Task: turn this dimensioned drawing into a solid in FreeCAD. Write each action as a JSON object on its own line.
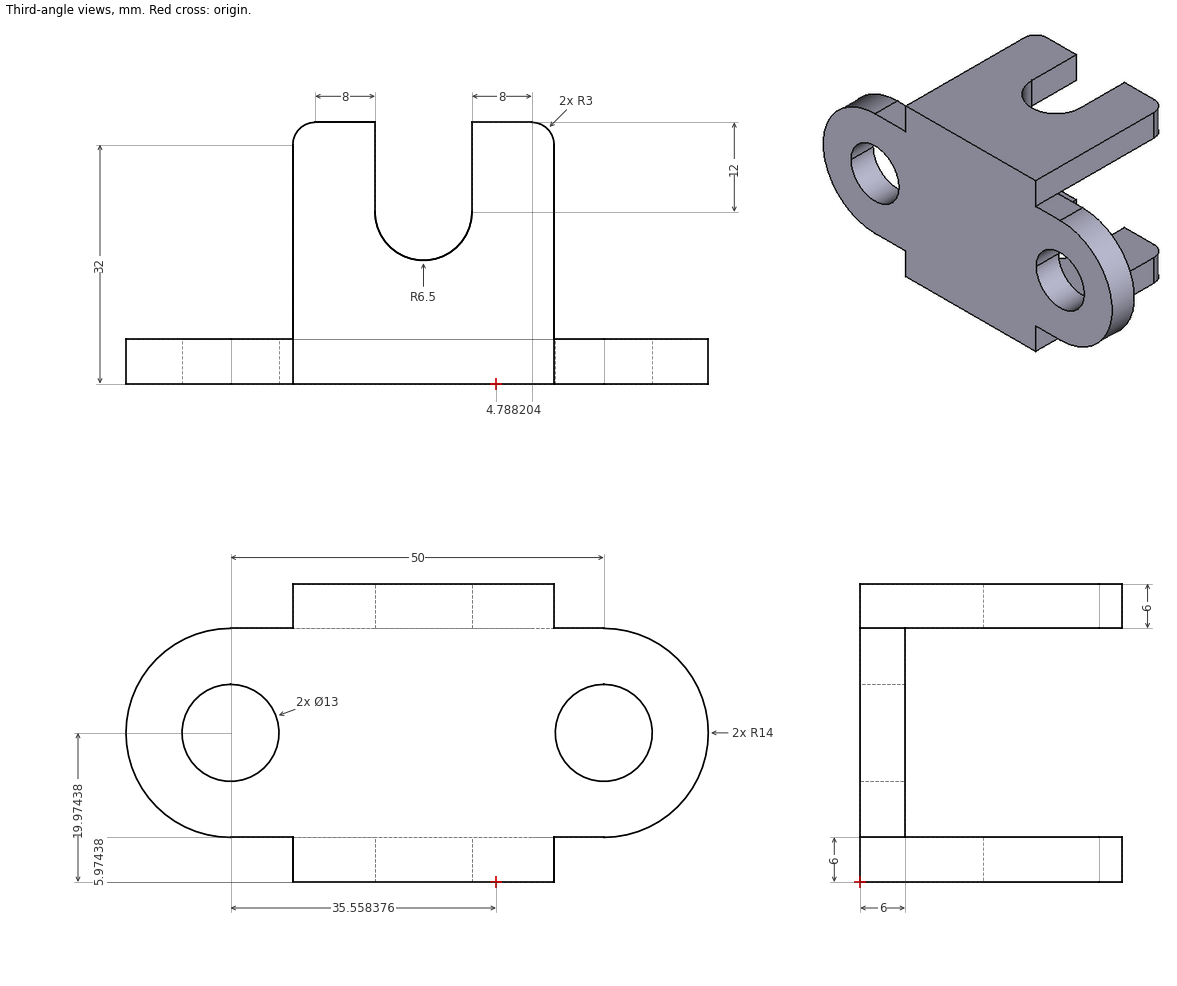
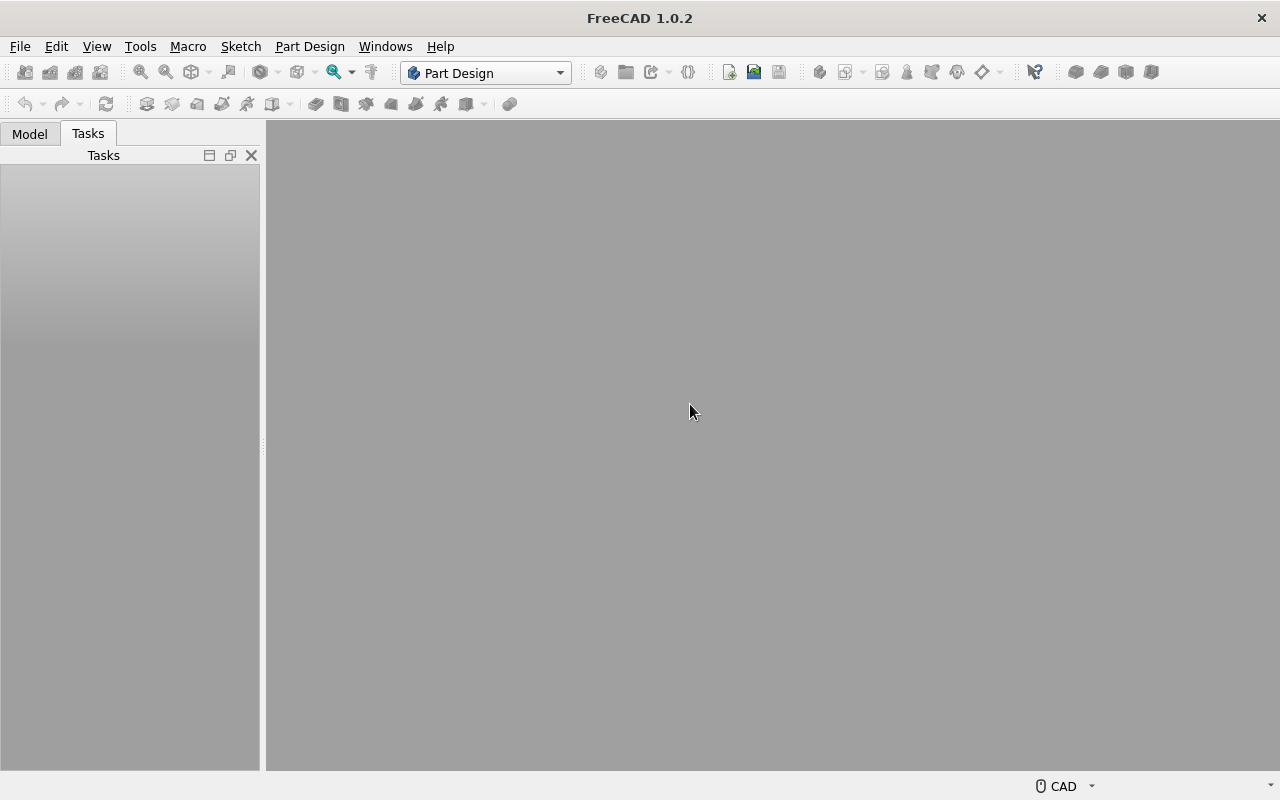
{"action": "left_click", "coordinate": [729, 72]}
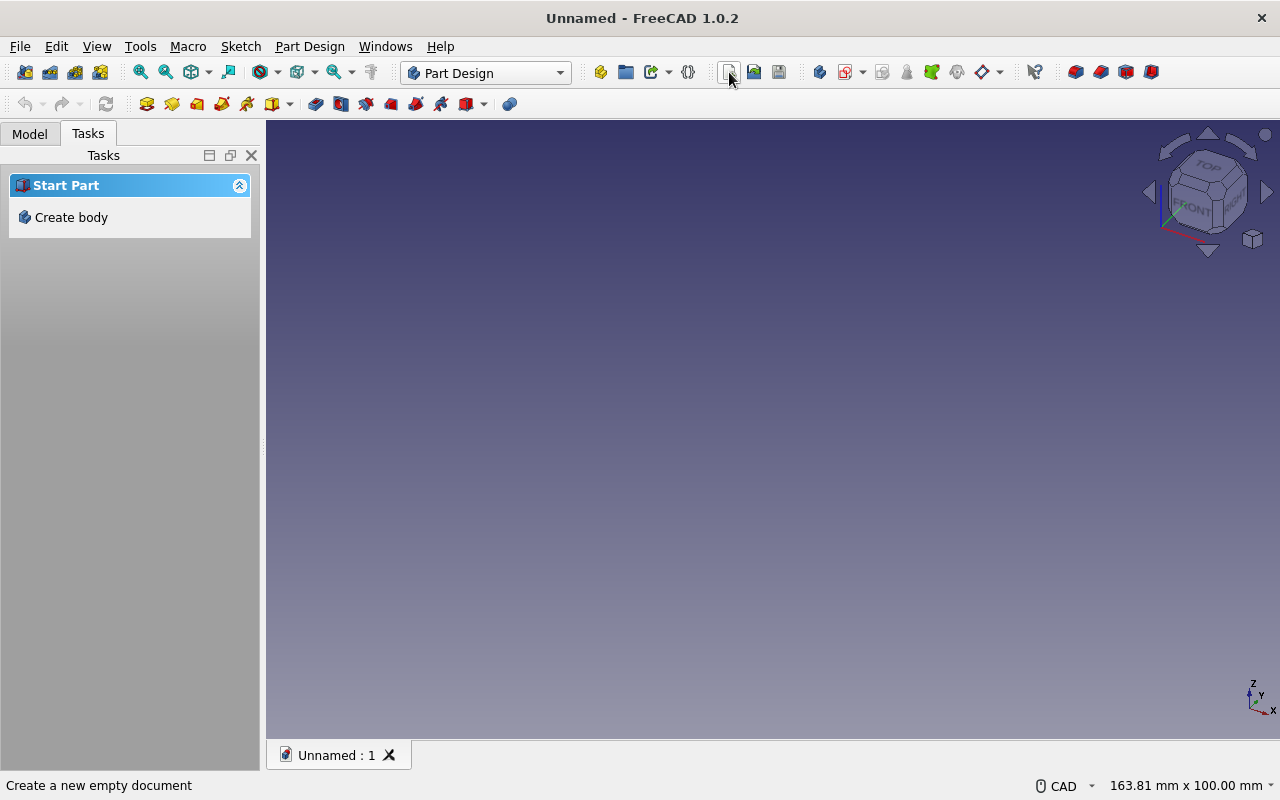
{"action": "left_click", "coordinate": [844, 72]}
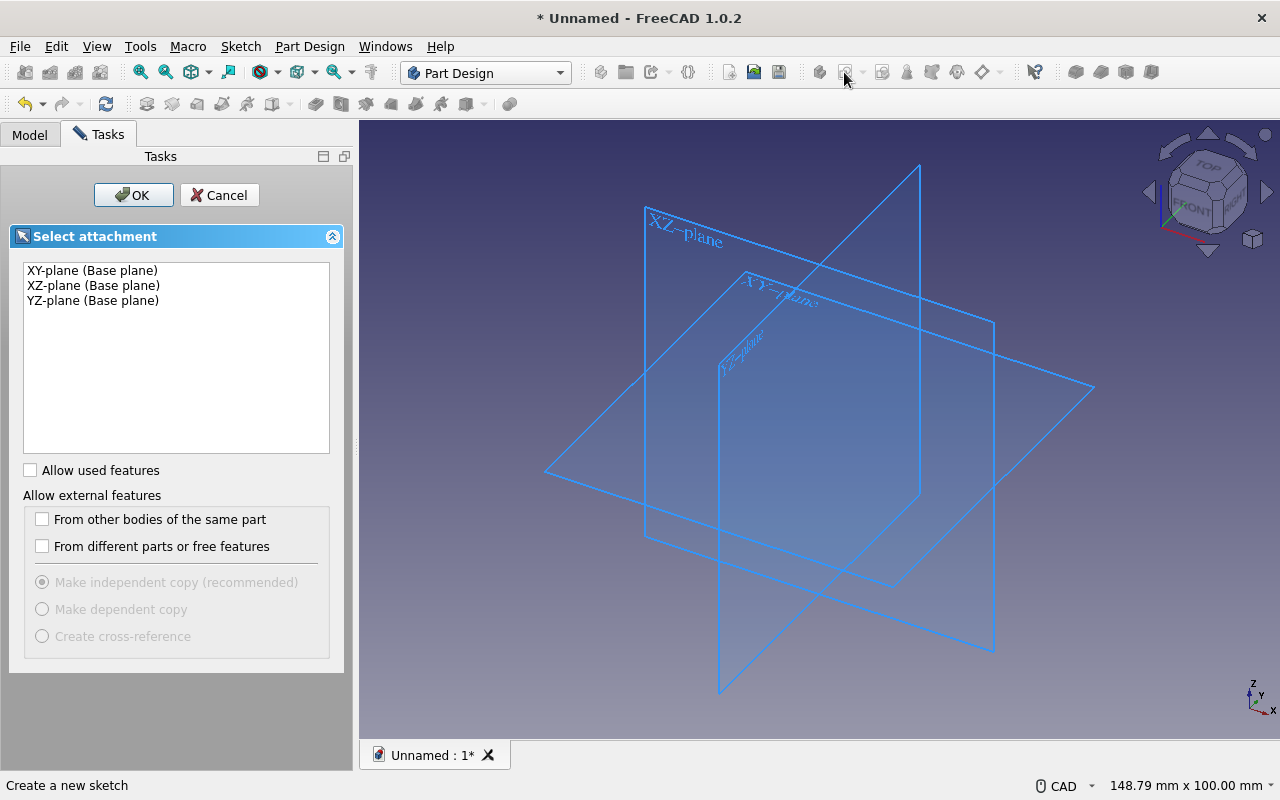
{"action": "left_click", "coordinate": [84, 270]}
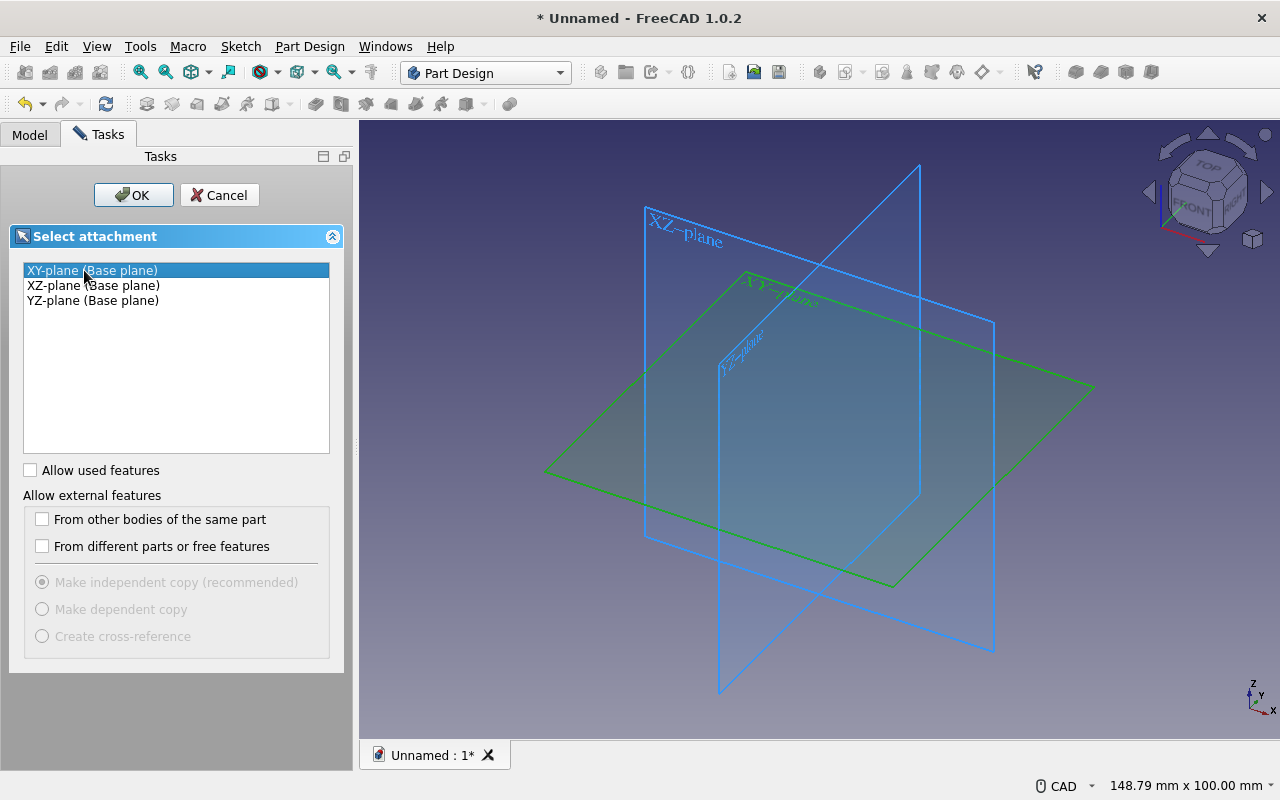
{"action": "left_click", "coordinate": [134, 195]}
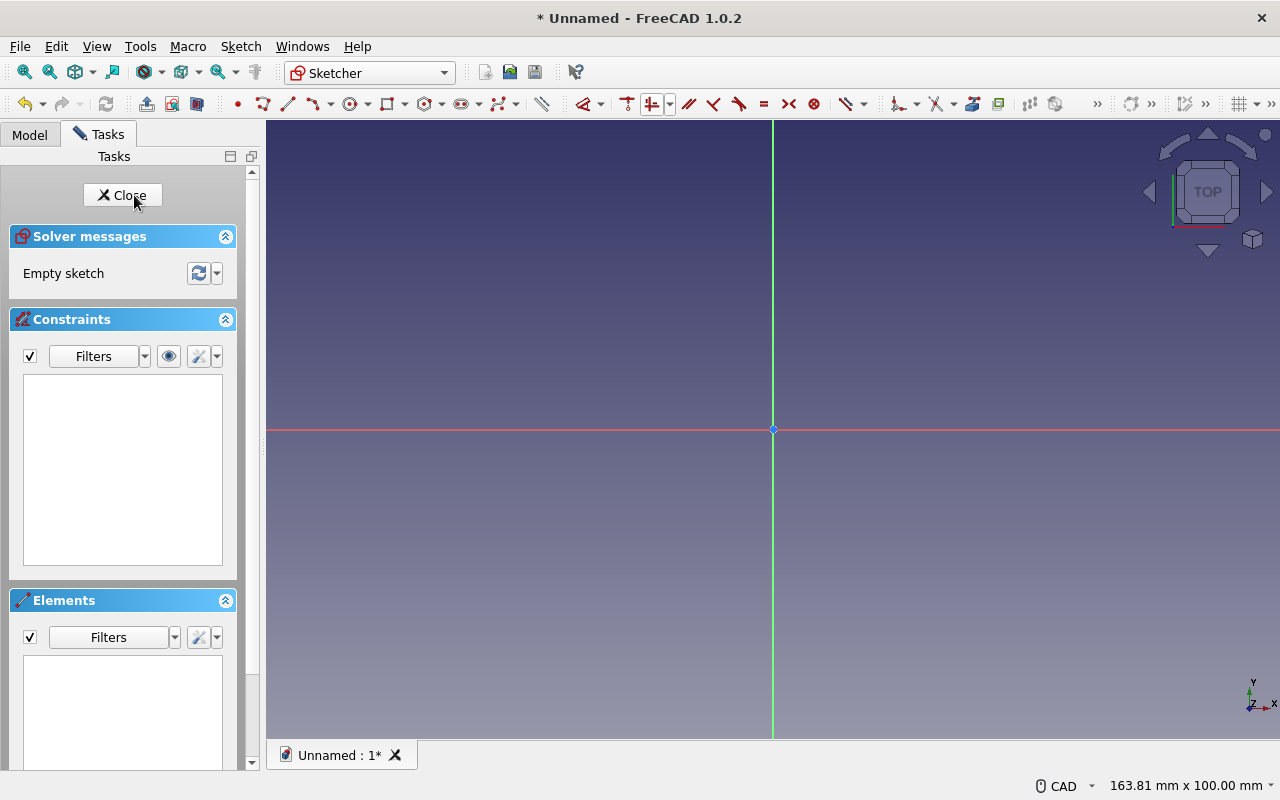
{"action": "scroll", "coordinate": [723, 189], "scroll_direction": "up", "scroll_amount": 3}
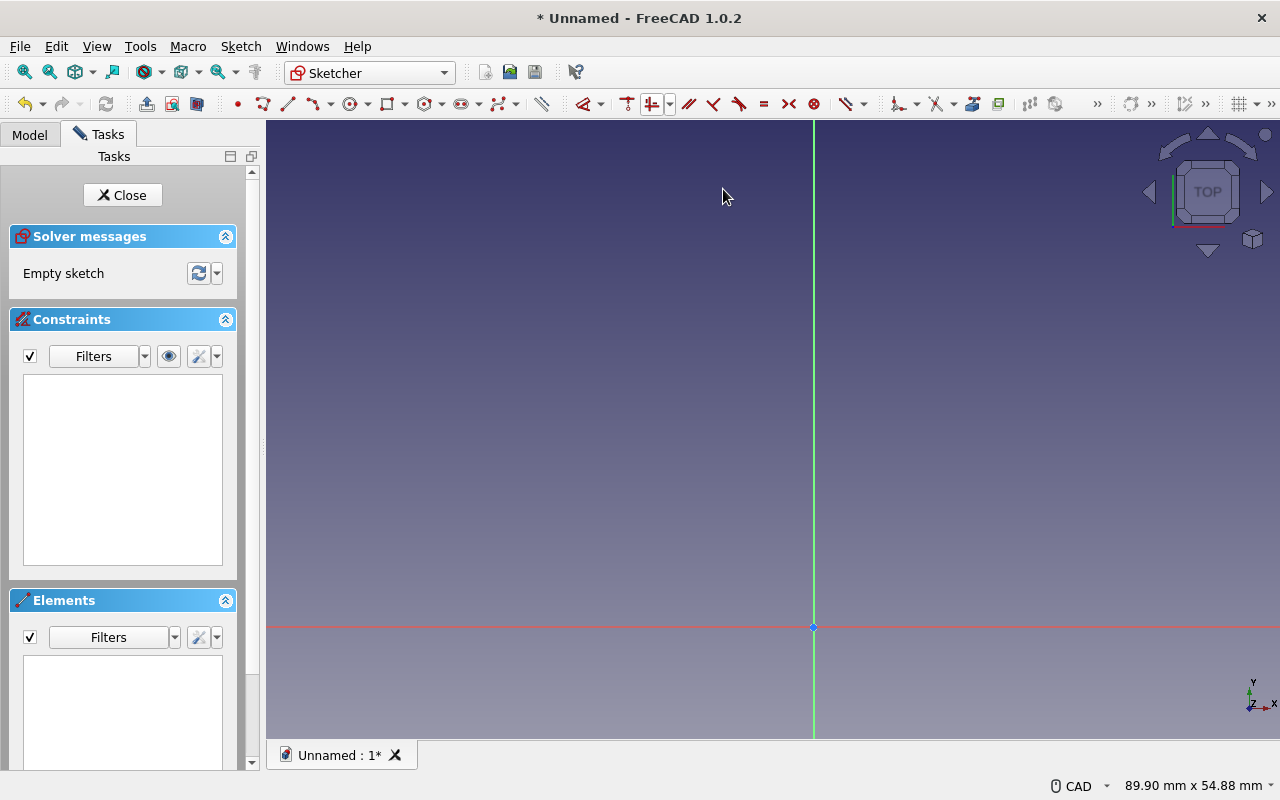
{"action": "left_click", "coordinate": [263, 104]}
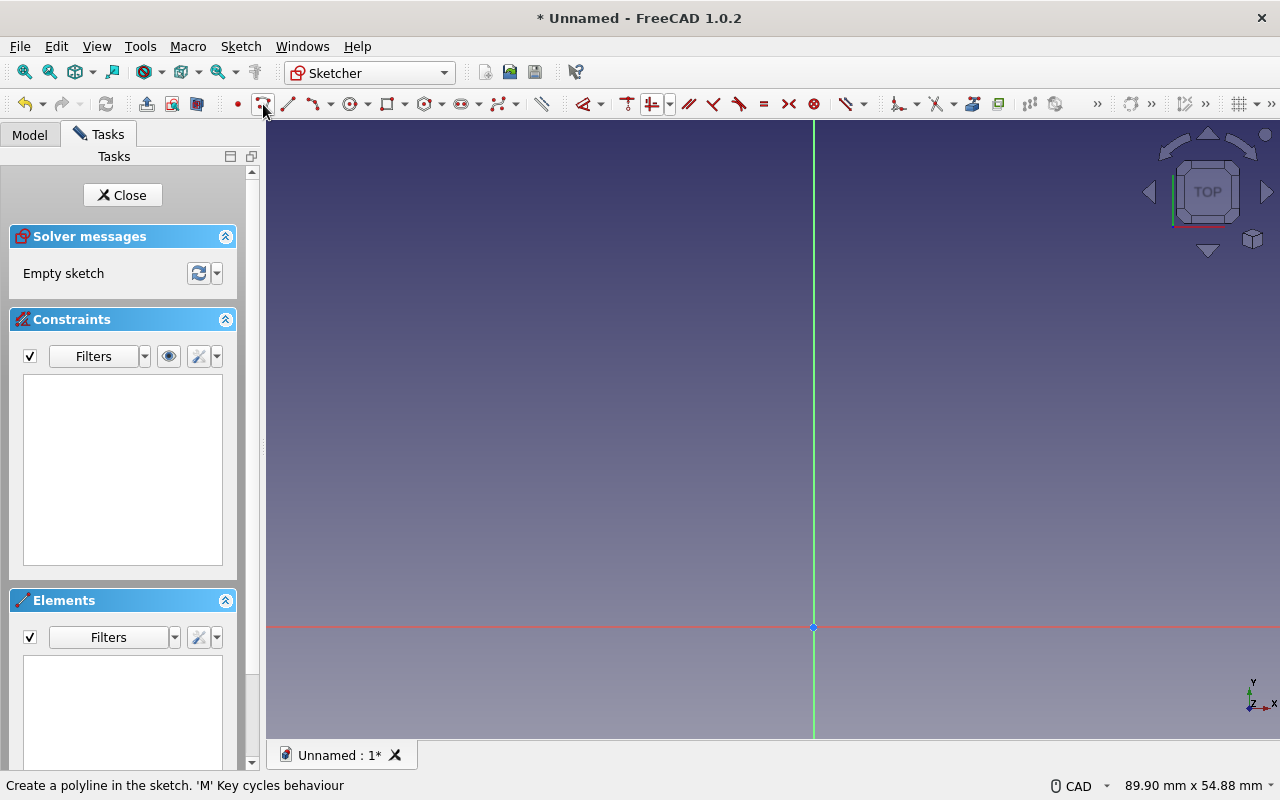
{"action": "left_click", "coordinate": [868, 232]}
{"action": "left_click", "coordinate": [778, 232]}
{"action": "left_click", "coordinate": [778, 368]}
{"action": "right_click", "coordinate": [778, 368]}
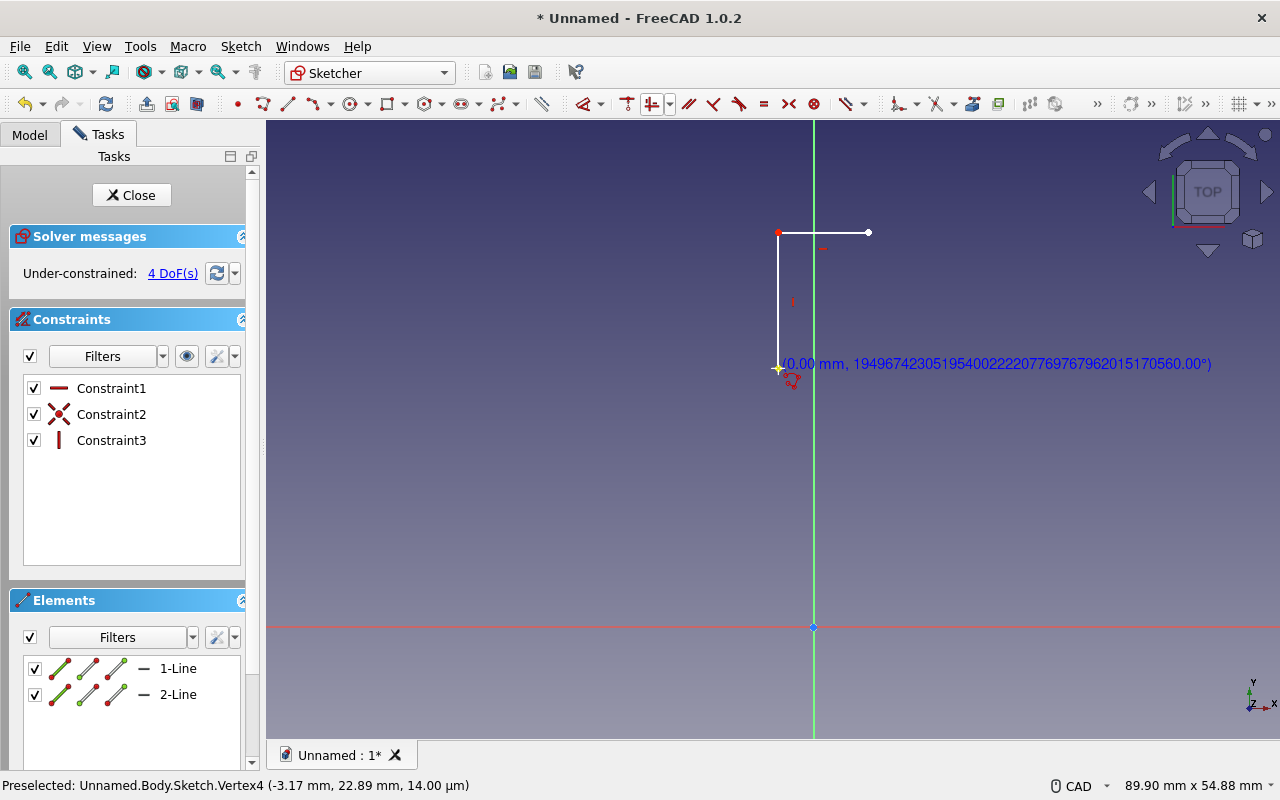
{"action": "left_click", "coordinate": [631, 368]}
{"action": "left_click", "coordinate": [631, 232]}
{"action": "left_click", "coordinate": [541, 232]}
{"action": "right_click", "coordinate": [541, 232]}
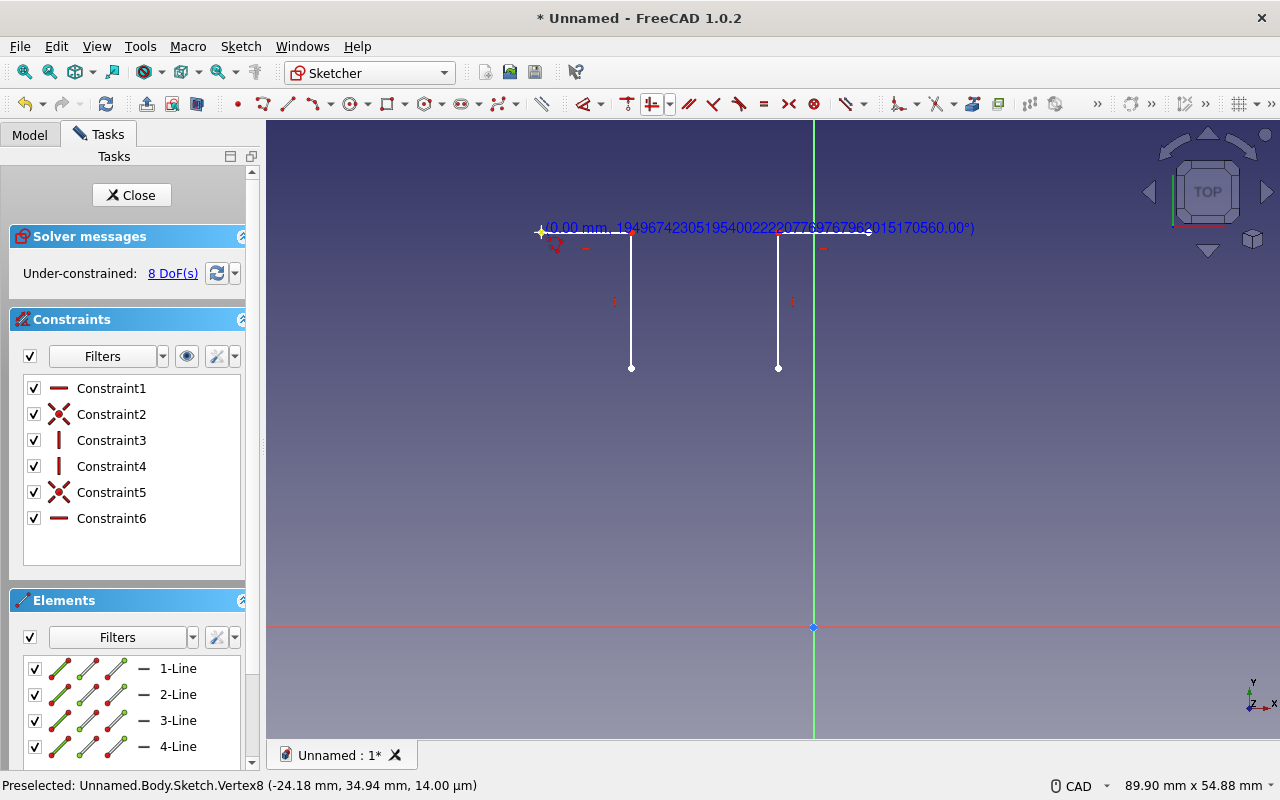
{"action": "left_click", "coordinate": [507, 266]}
{"action": "left_click", "coordinate": [507, 627]}
{"action": "left_click", "coordinate": [902, 618]}
{"action": "left_click", "coordinate": [902, 266]}
{"action": "right_click", "coordinate": [902, 266]}